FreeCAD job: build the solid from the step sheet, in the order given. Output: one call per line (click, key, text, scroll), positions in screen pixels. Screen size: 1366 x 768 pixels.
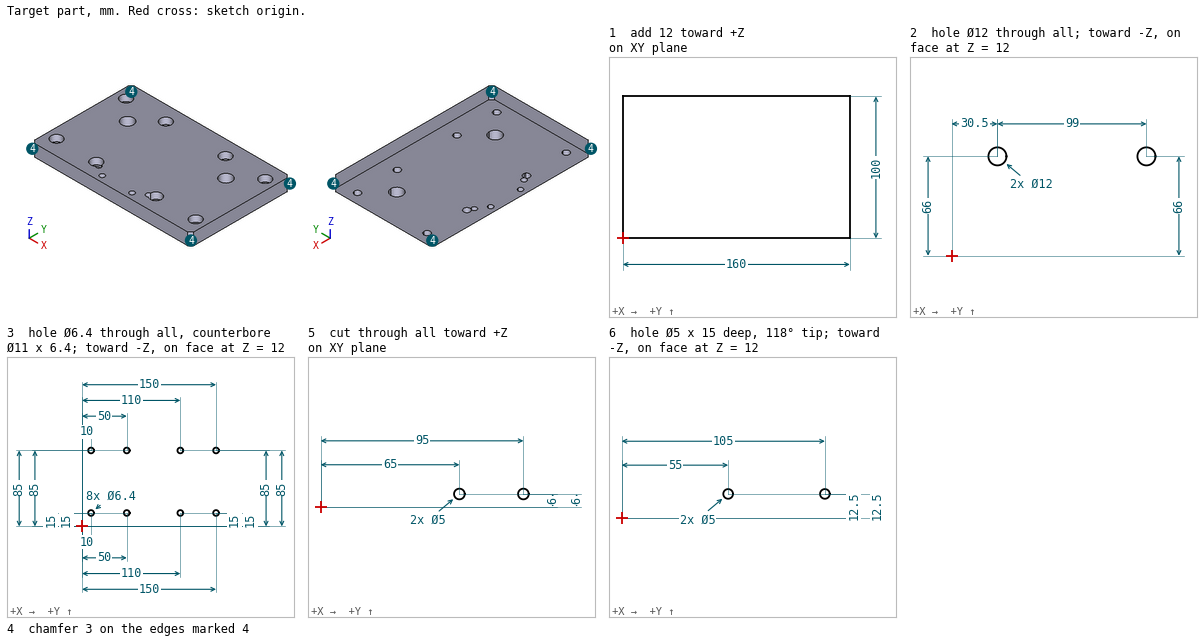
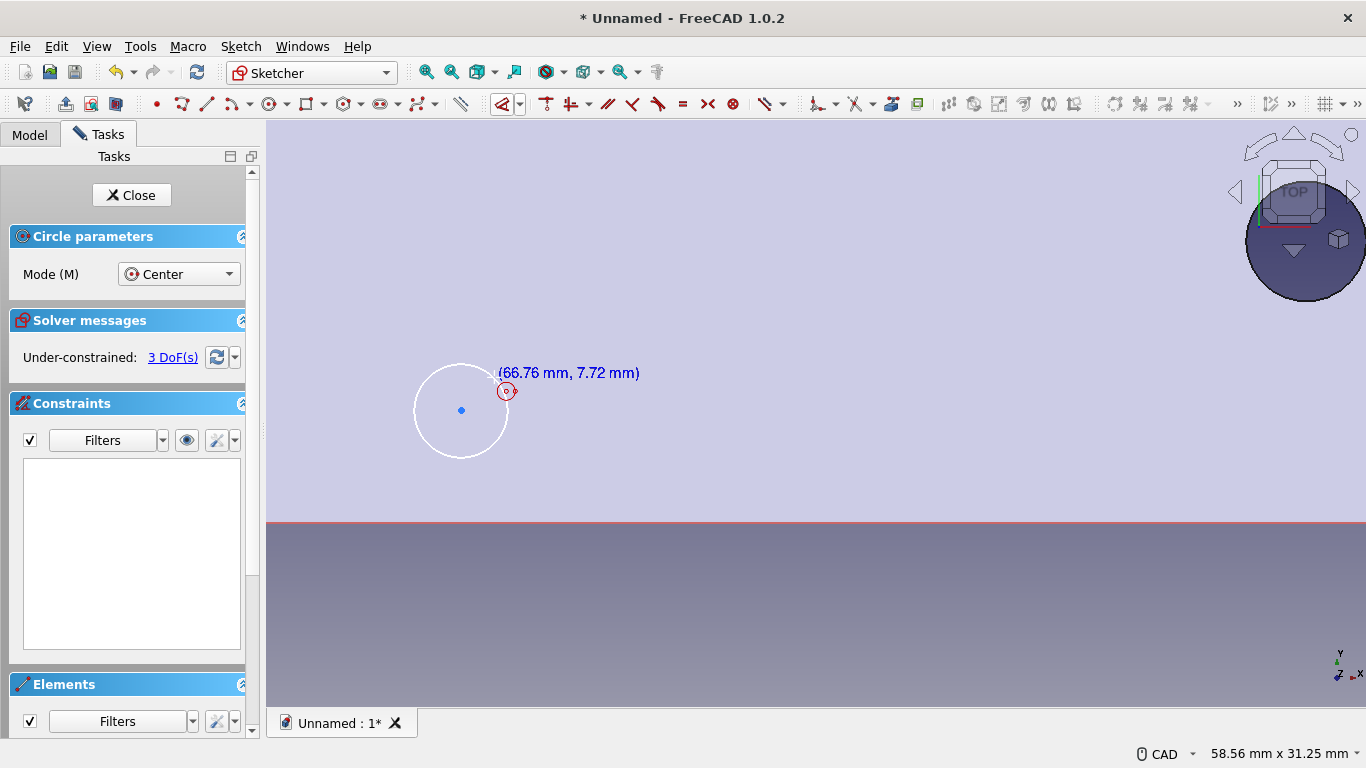
click(1024, 410)
click(1058, 377)
key(Escape)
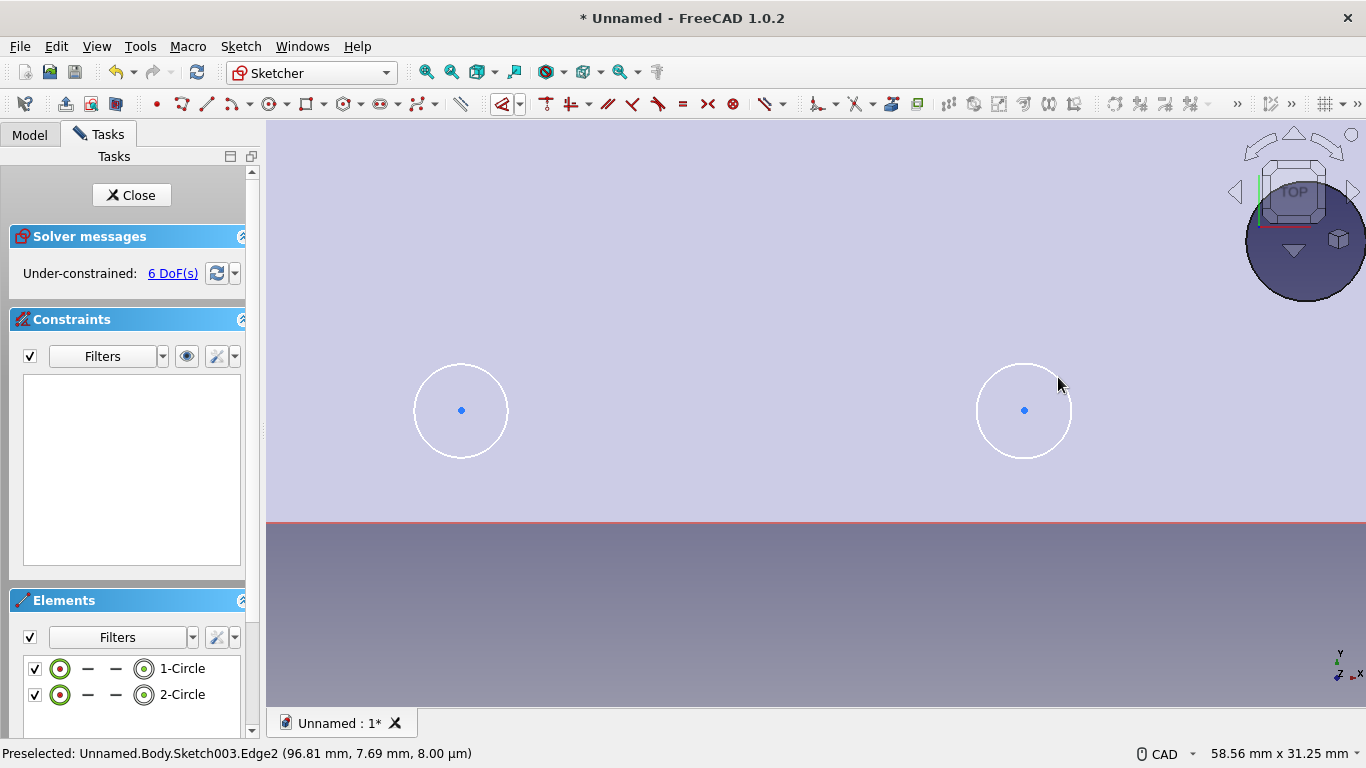
click(494, 378)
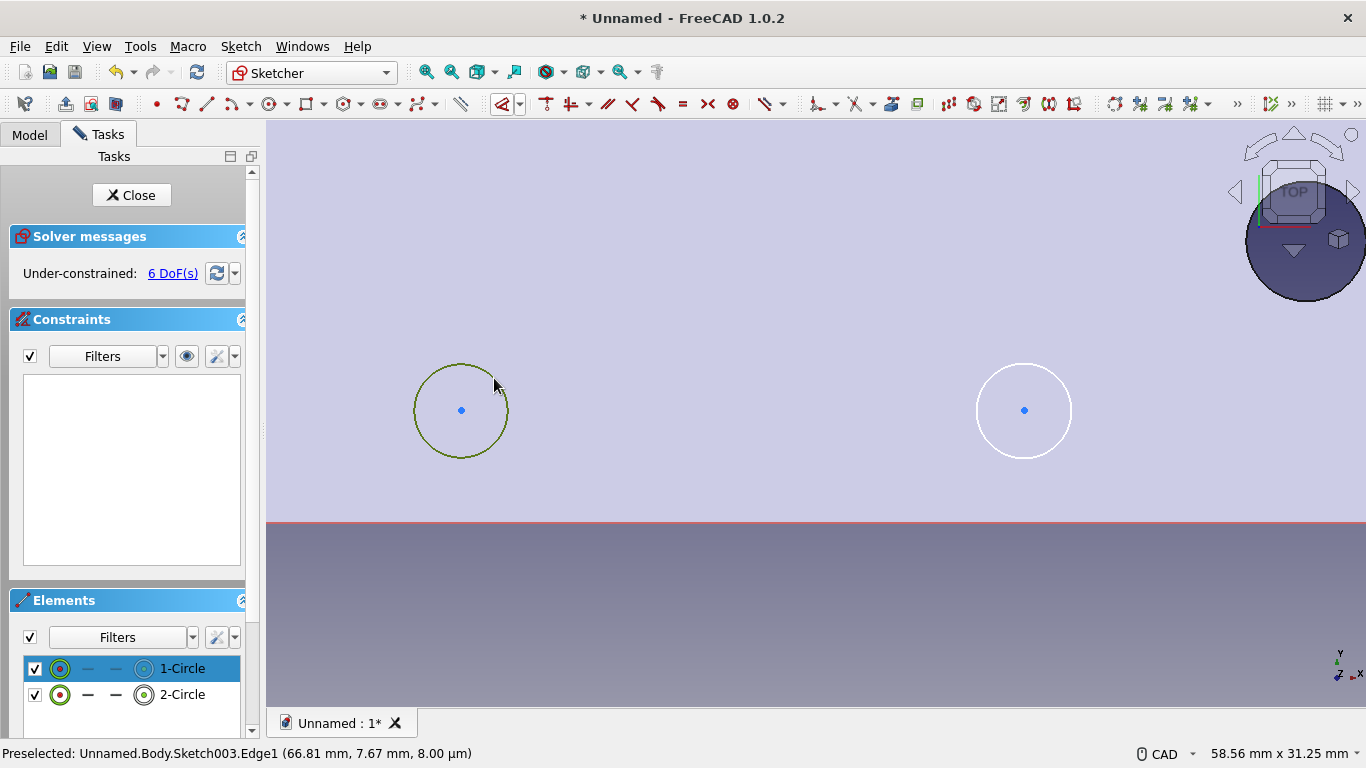
click(1057, 377)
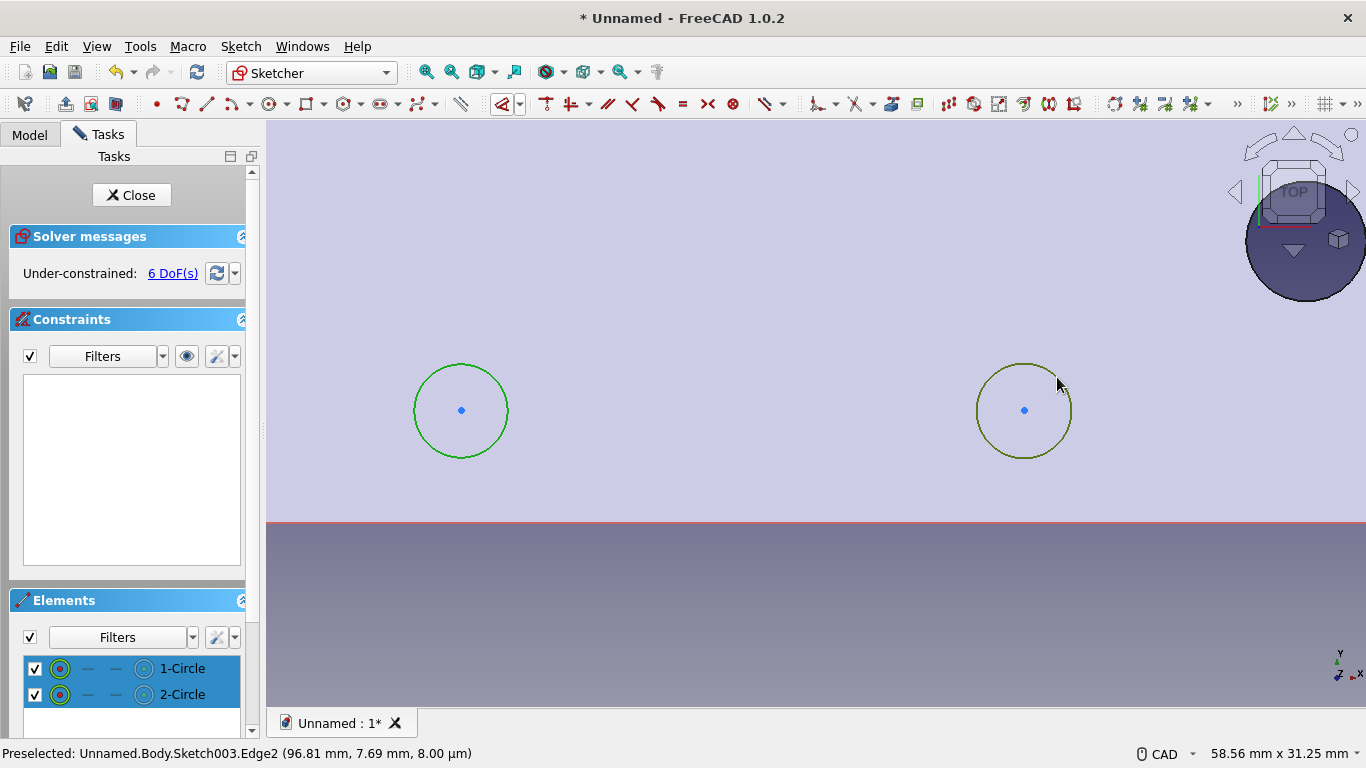
click(683, 104)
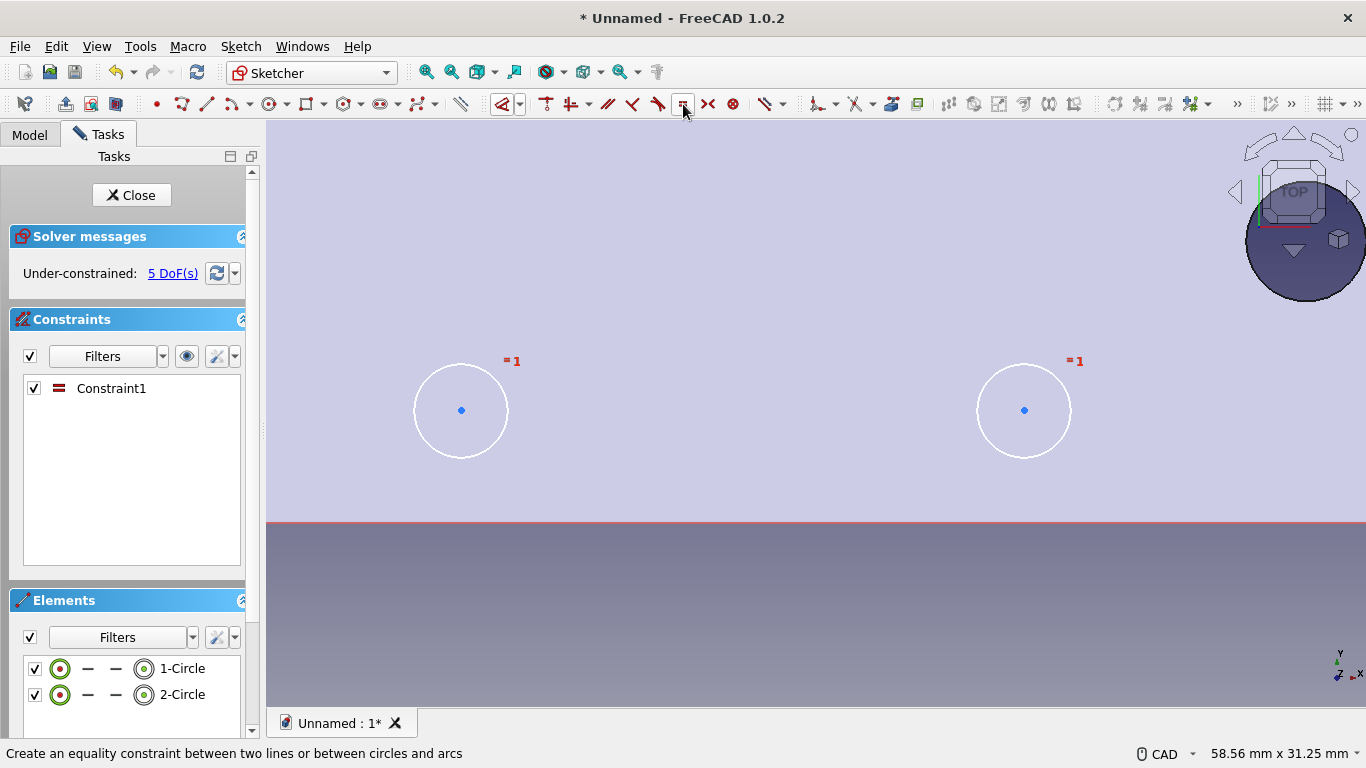
click(494, 378)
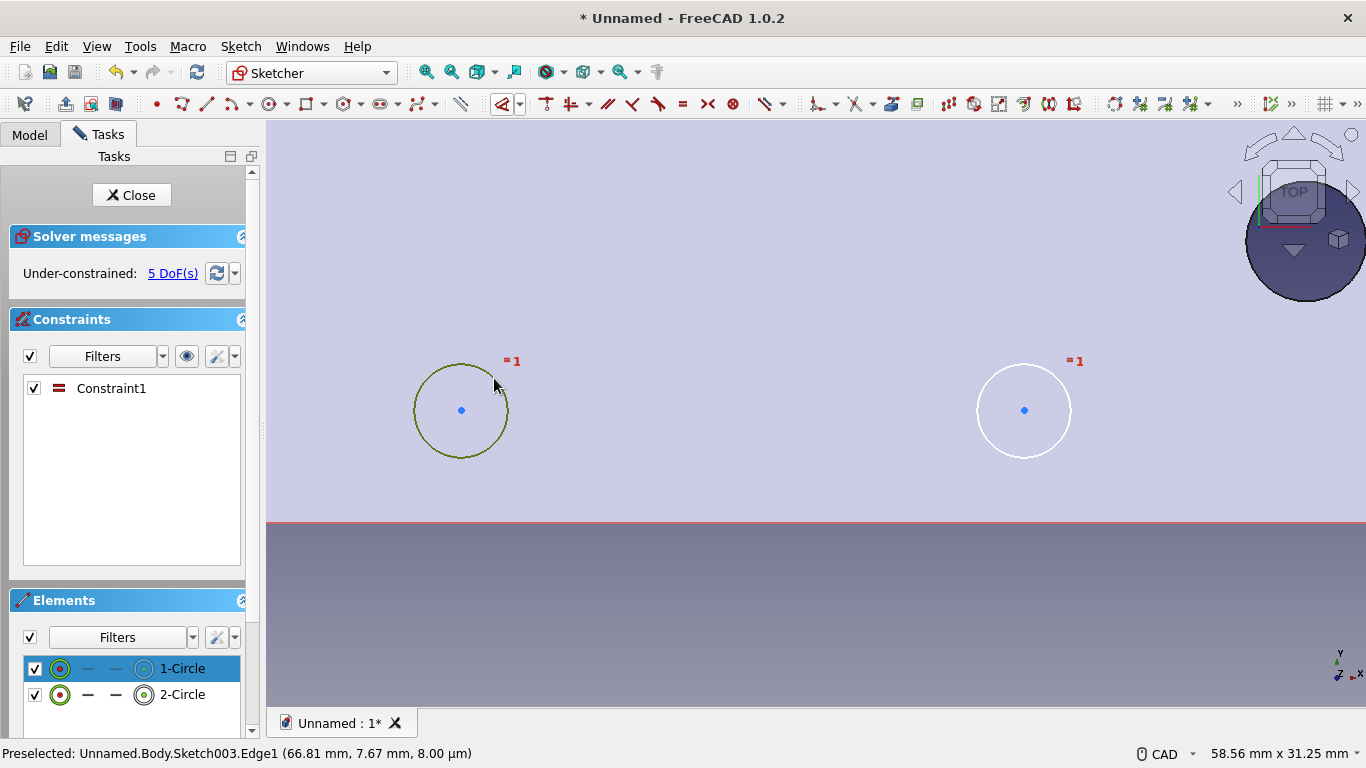
key(k)
key(o)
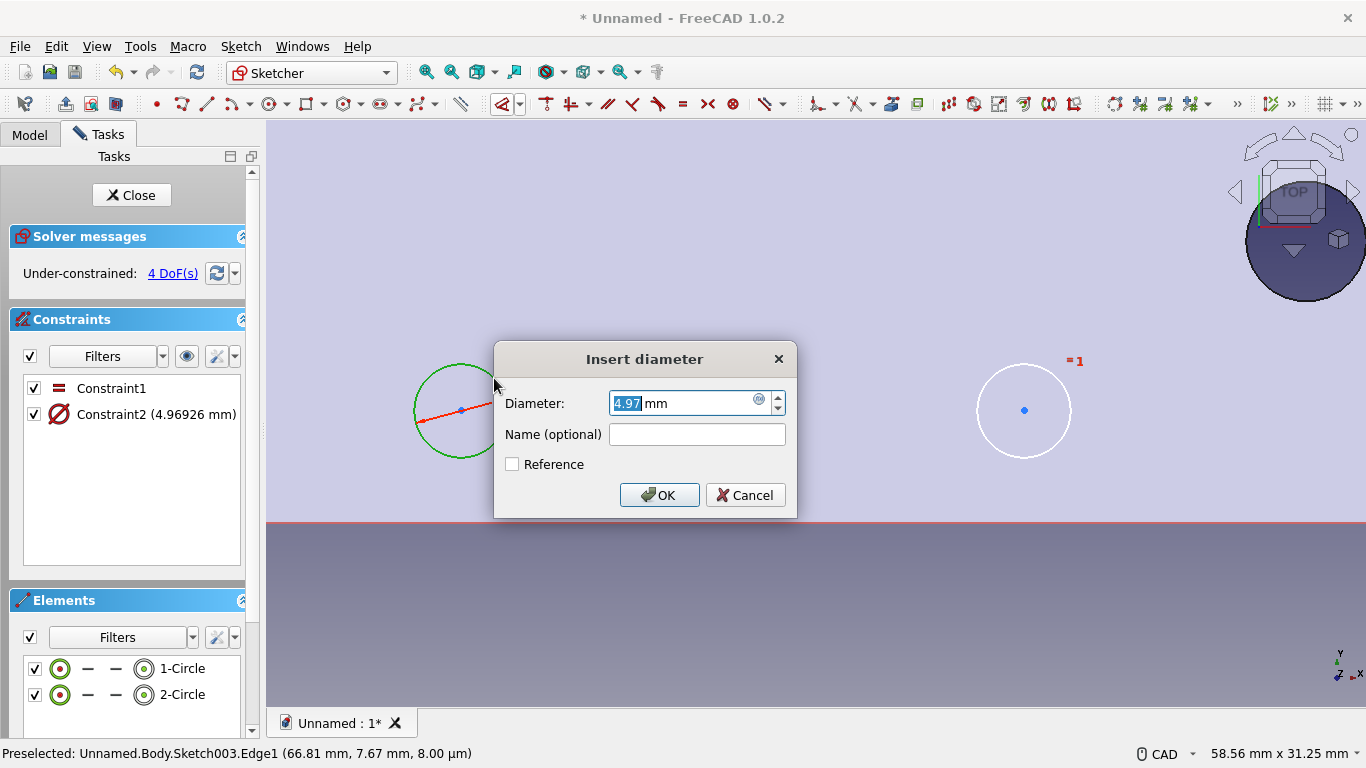
text(5)
key(Return)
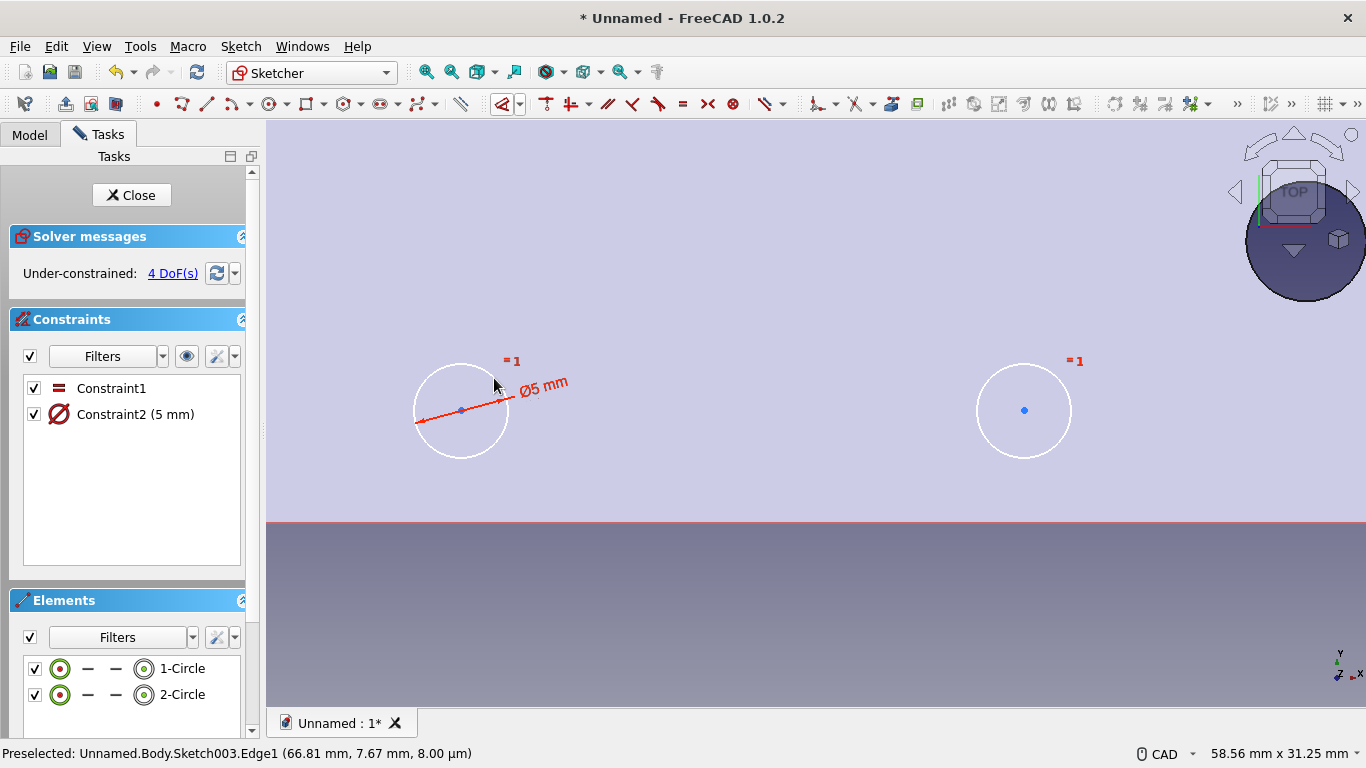
click(461, 411)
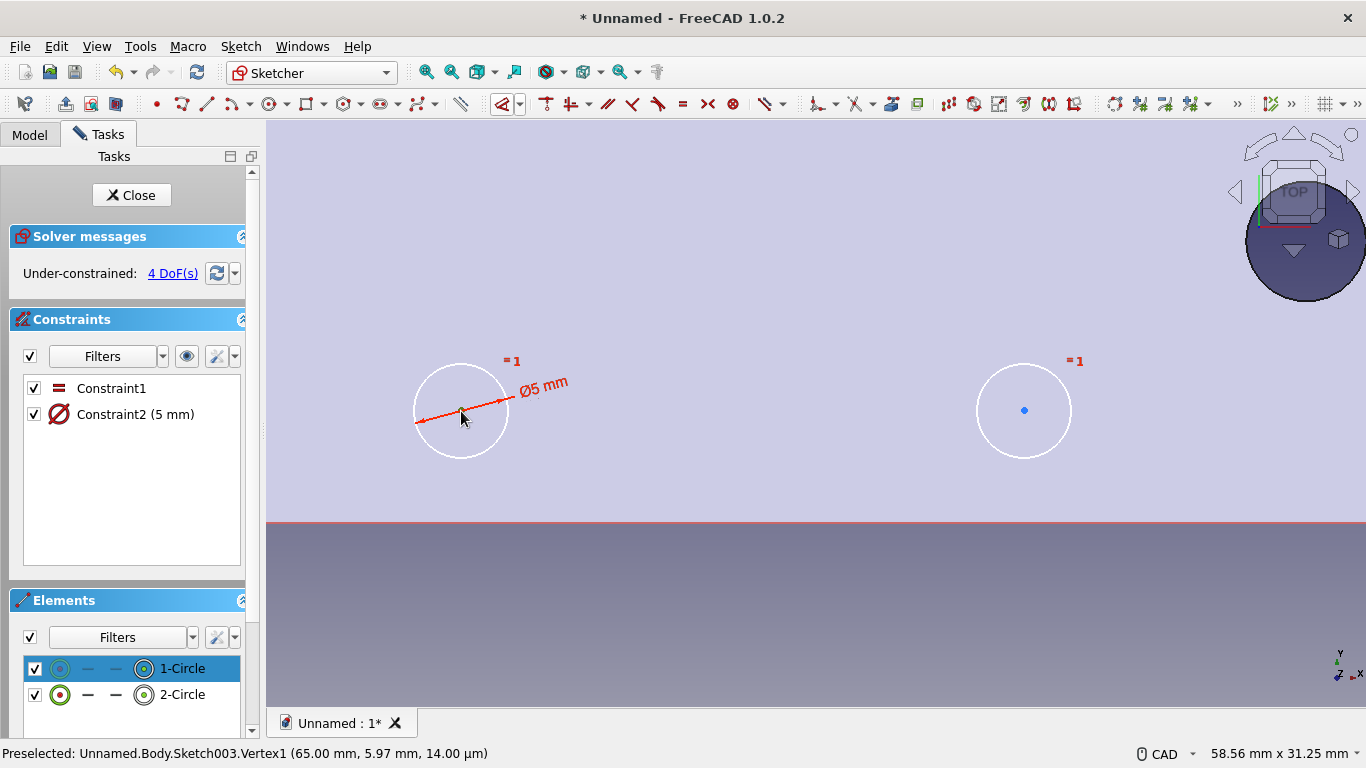
key(i)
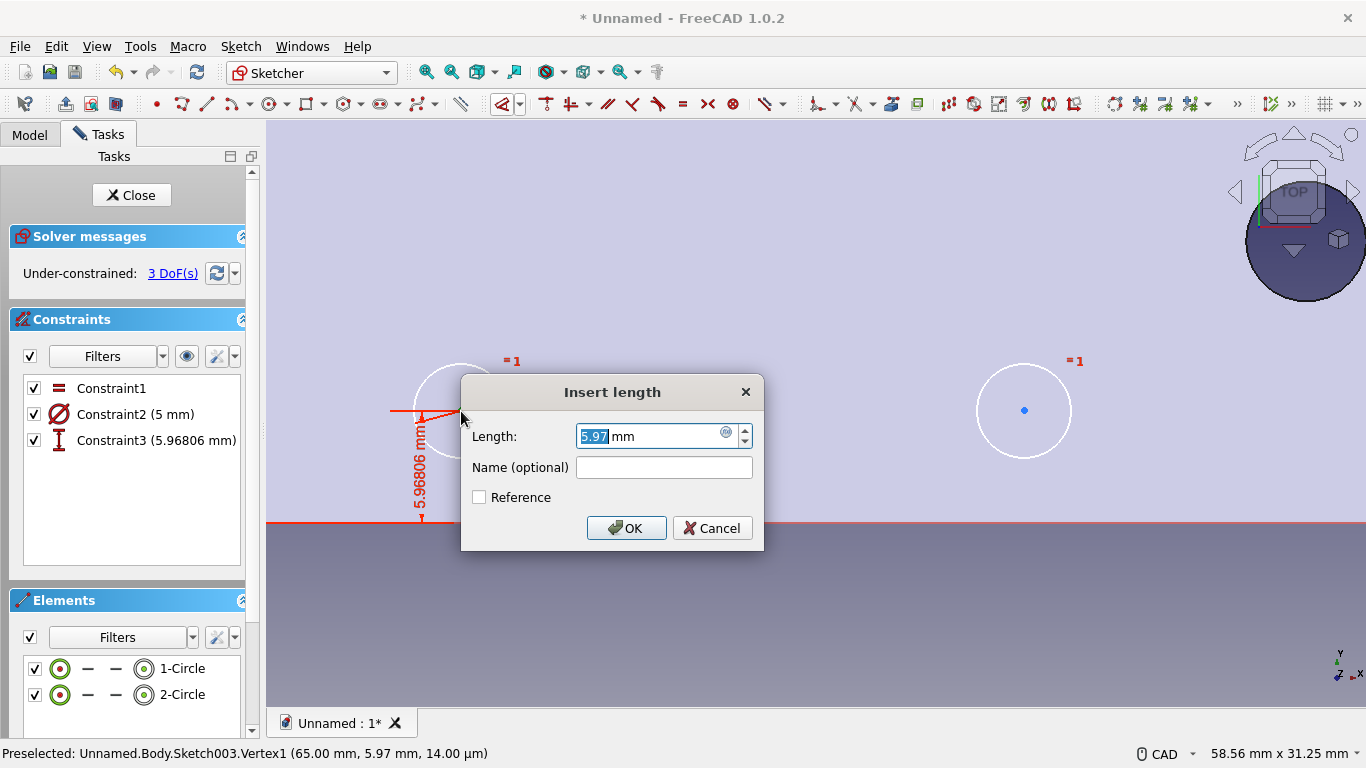
text(6)
key(Return)